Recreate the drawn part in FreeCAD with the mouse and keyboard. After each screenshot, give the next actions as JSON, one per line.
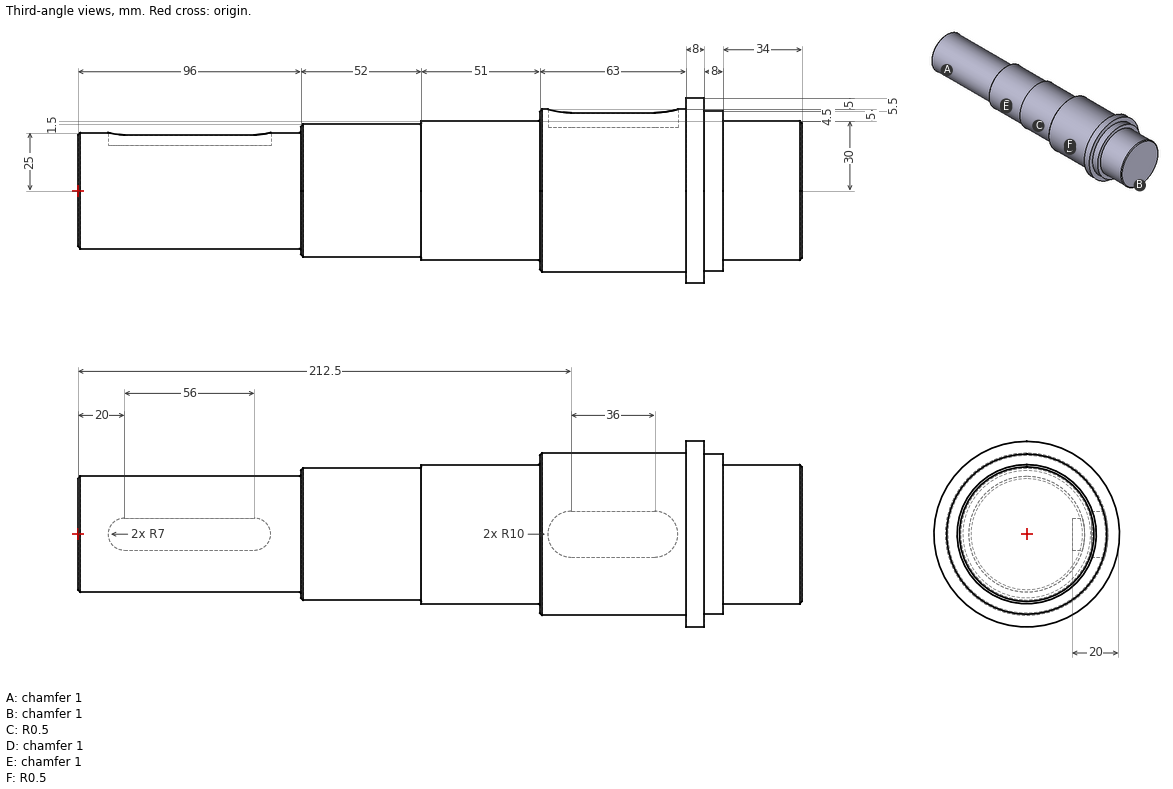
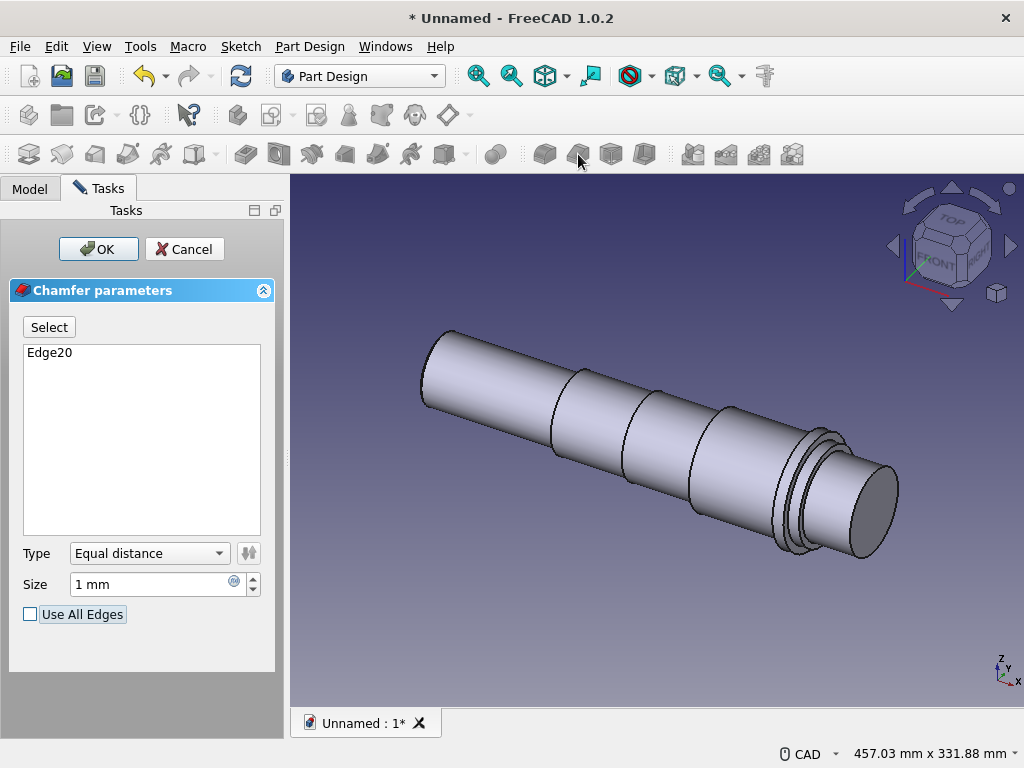
{"action": "left_click", "coordinate": [99, 249]}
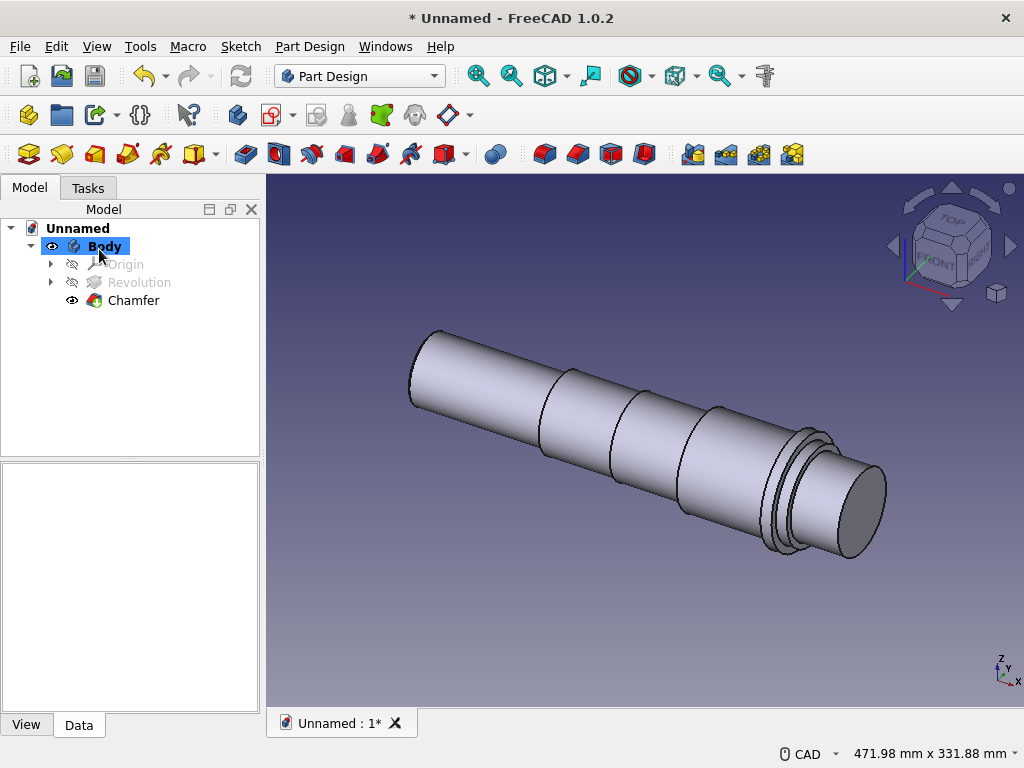
{"action": "left_click", "coordinate": [838, 535]}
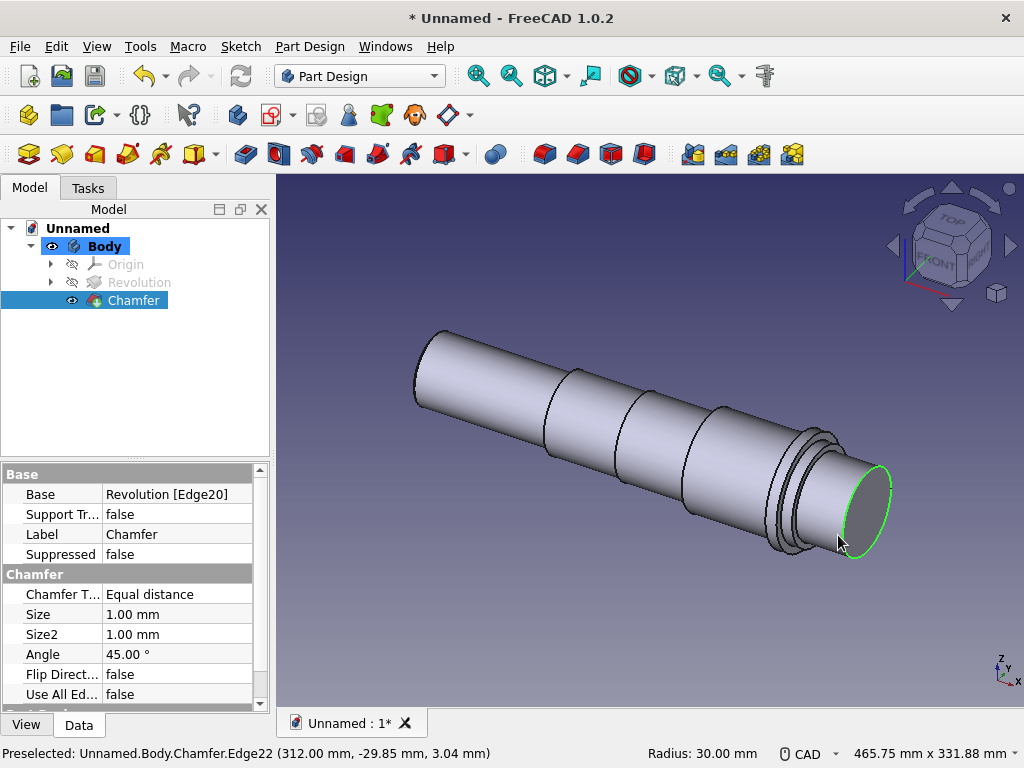
{"action": "left_click", "coordinate": [578, 154]}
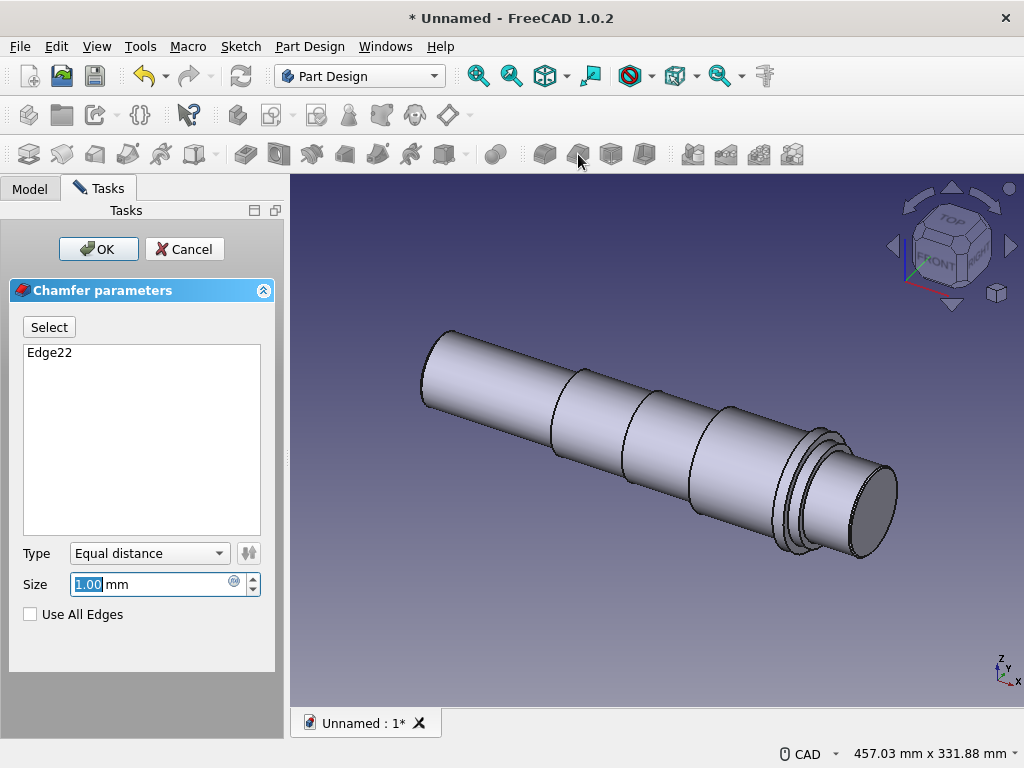
{"action": "type", "text": "1"}
{"action": "key", "text": "Tab"}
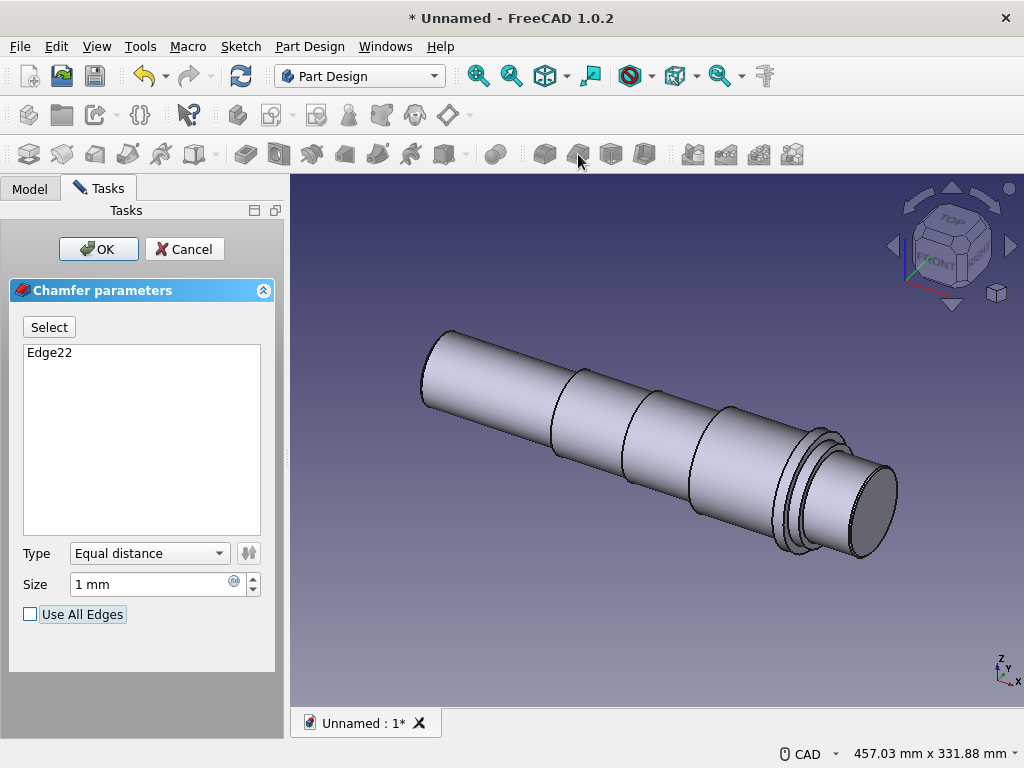
{"action": "left_click", "coordinate": [99, 249]}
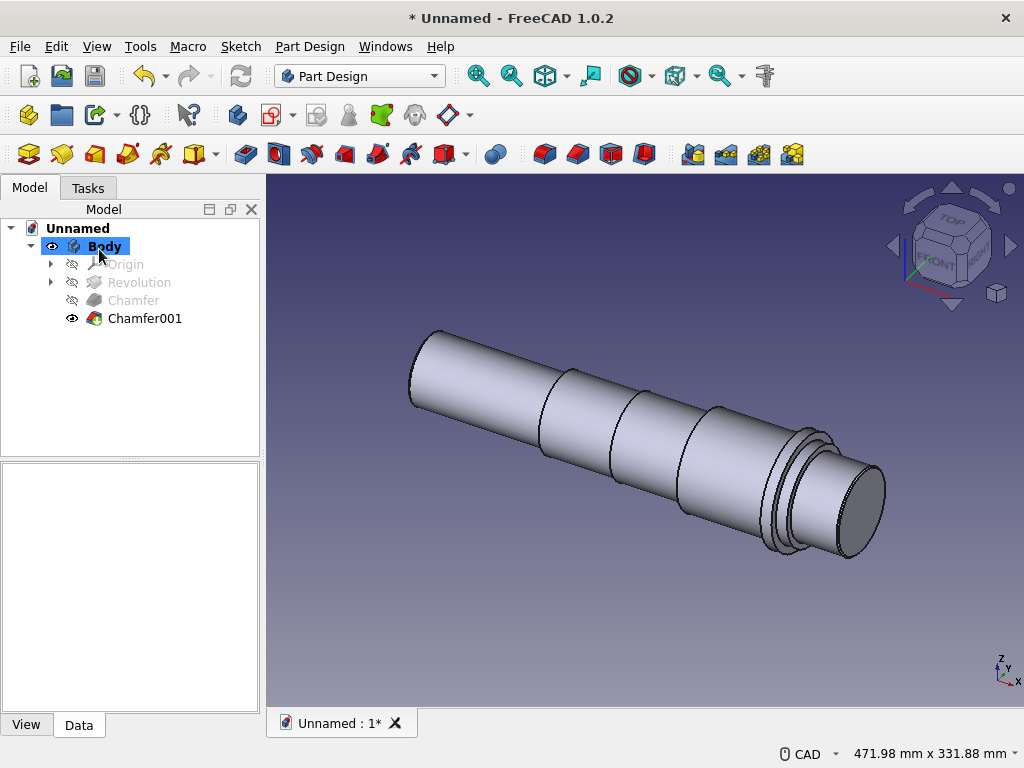
{"action": "key", "text": "0"}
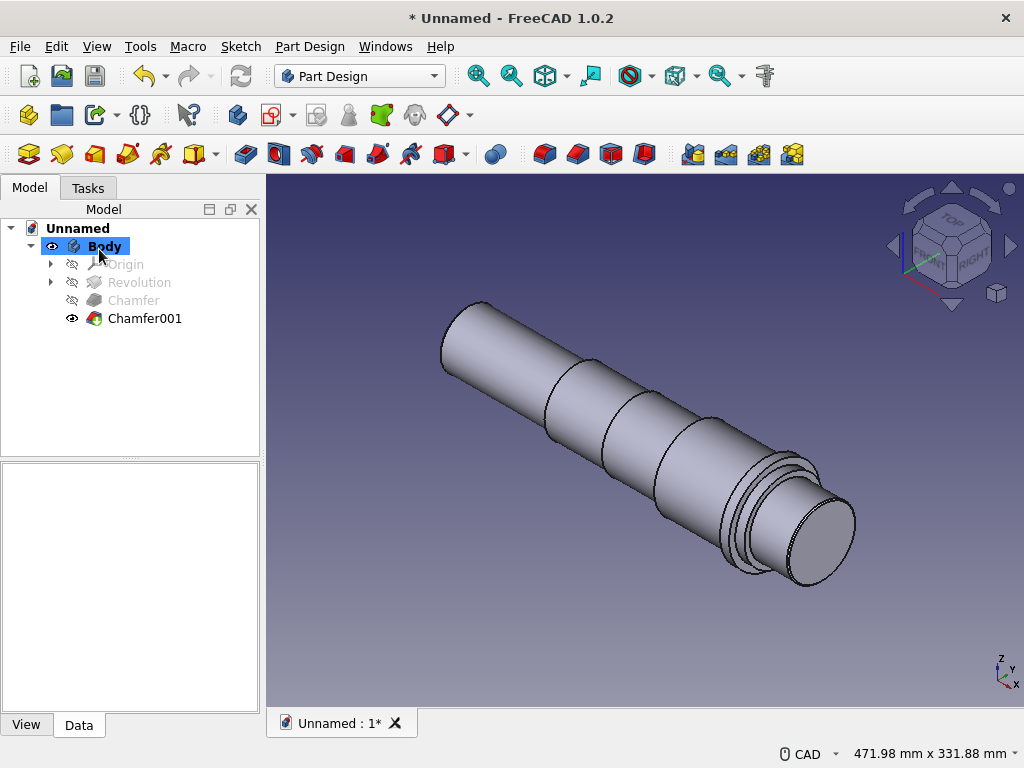
{"action": "key", "text": "2"}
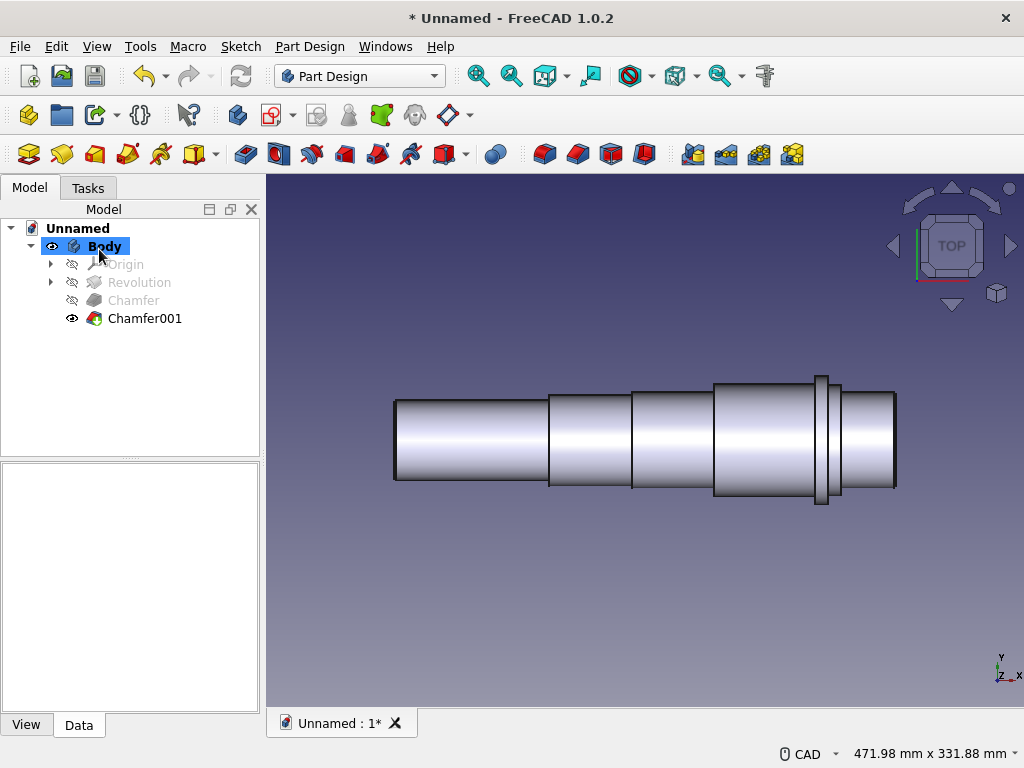
{"action": "key", "text": "1"}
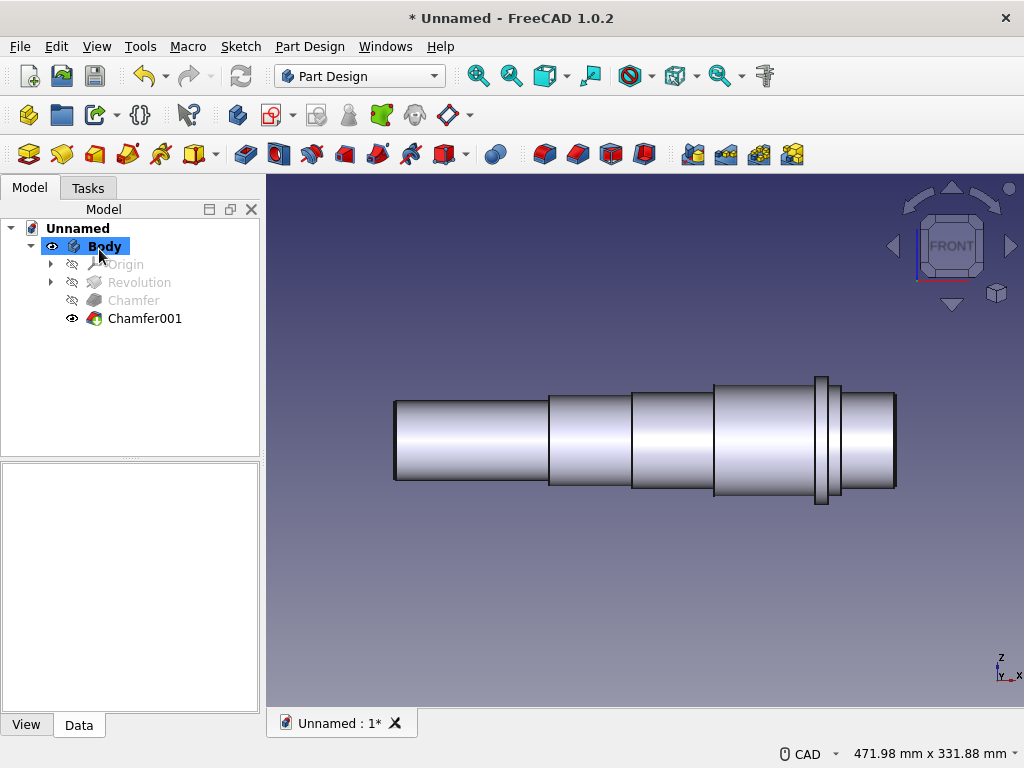
{"action": "key", "text": "3"}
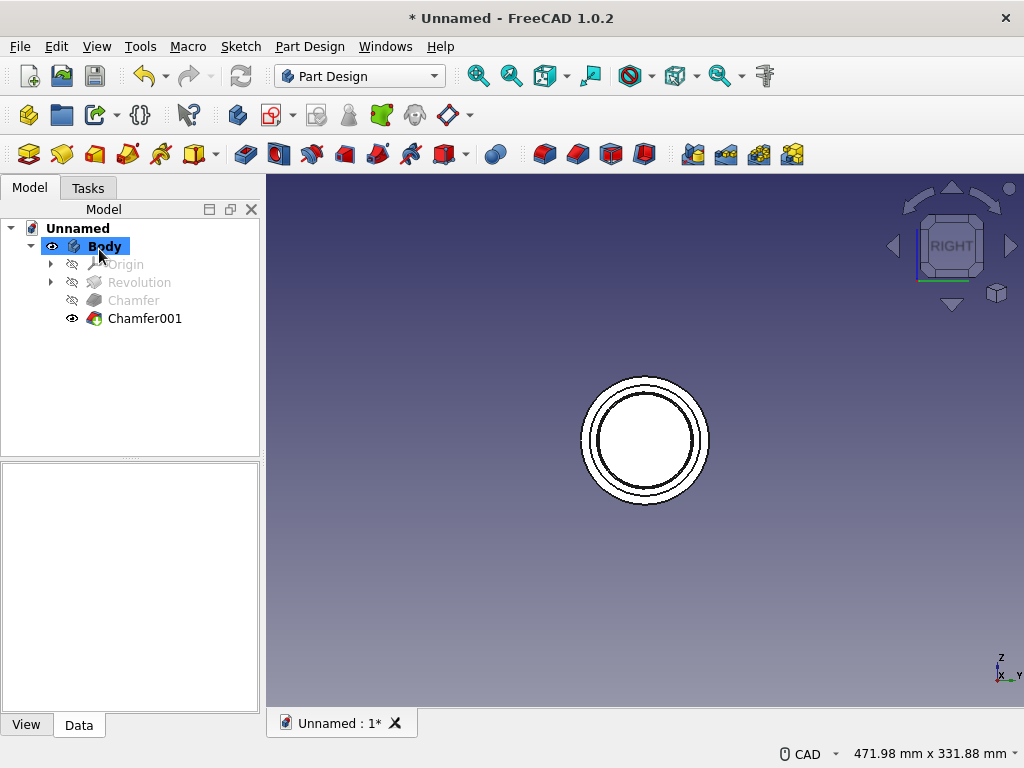
{"action": "key", "text": "v f"}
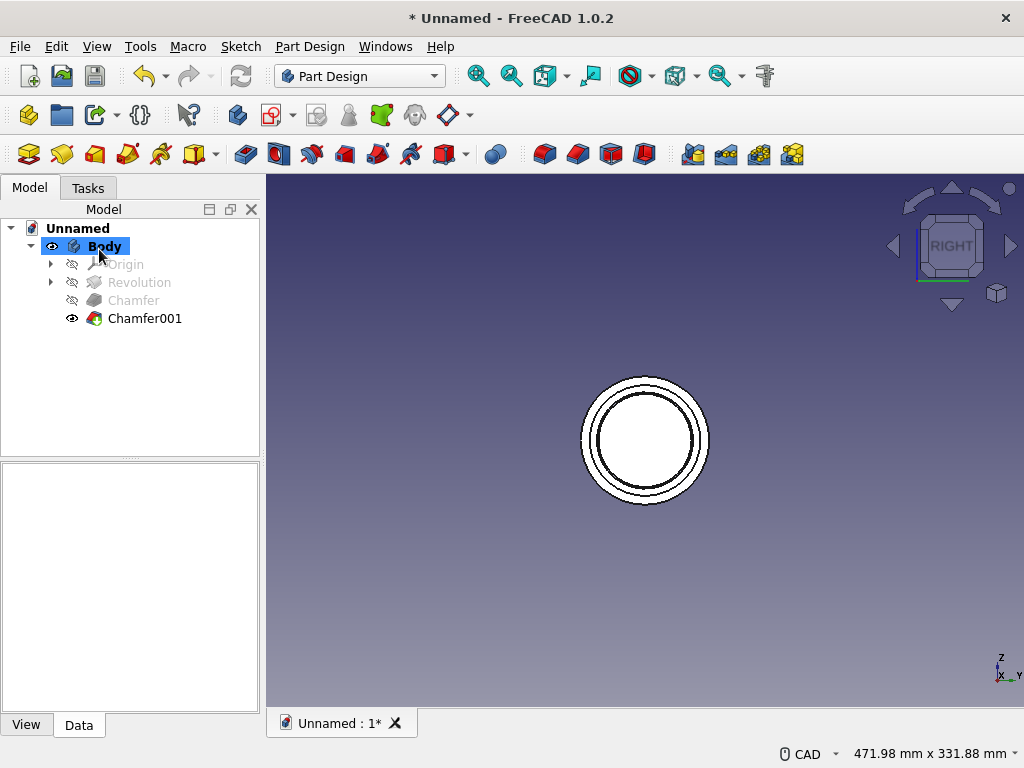
{"action": "key", "text": "5"}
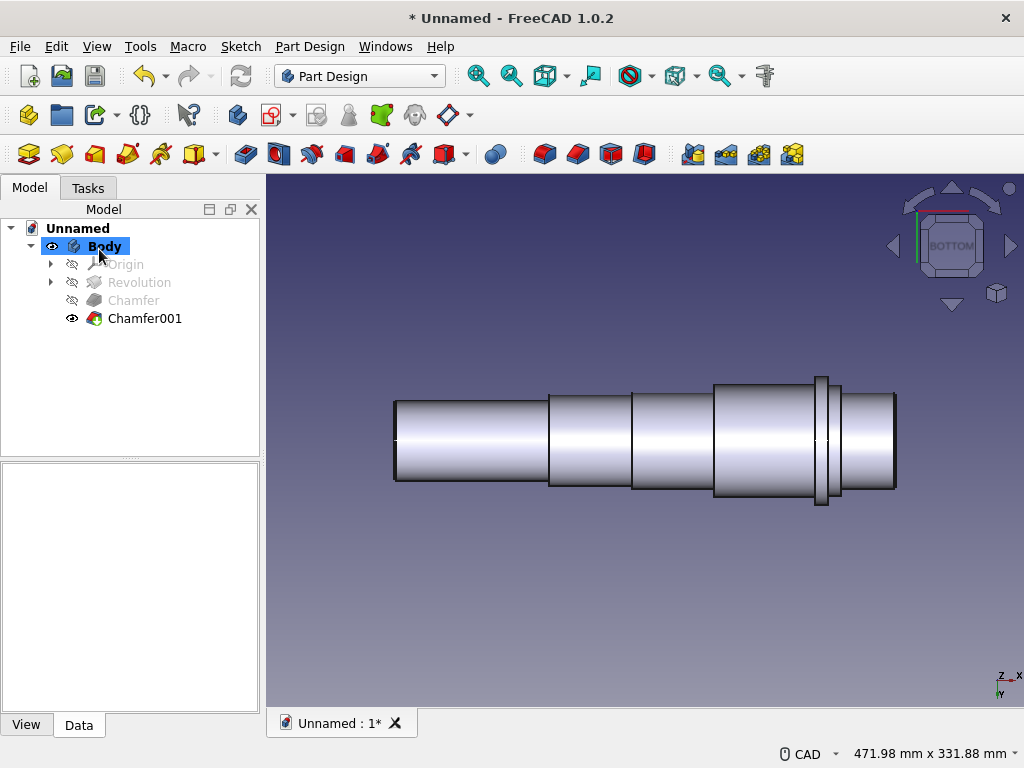
{"action": "key", "text": "4"}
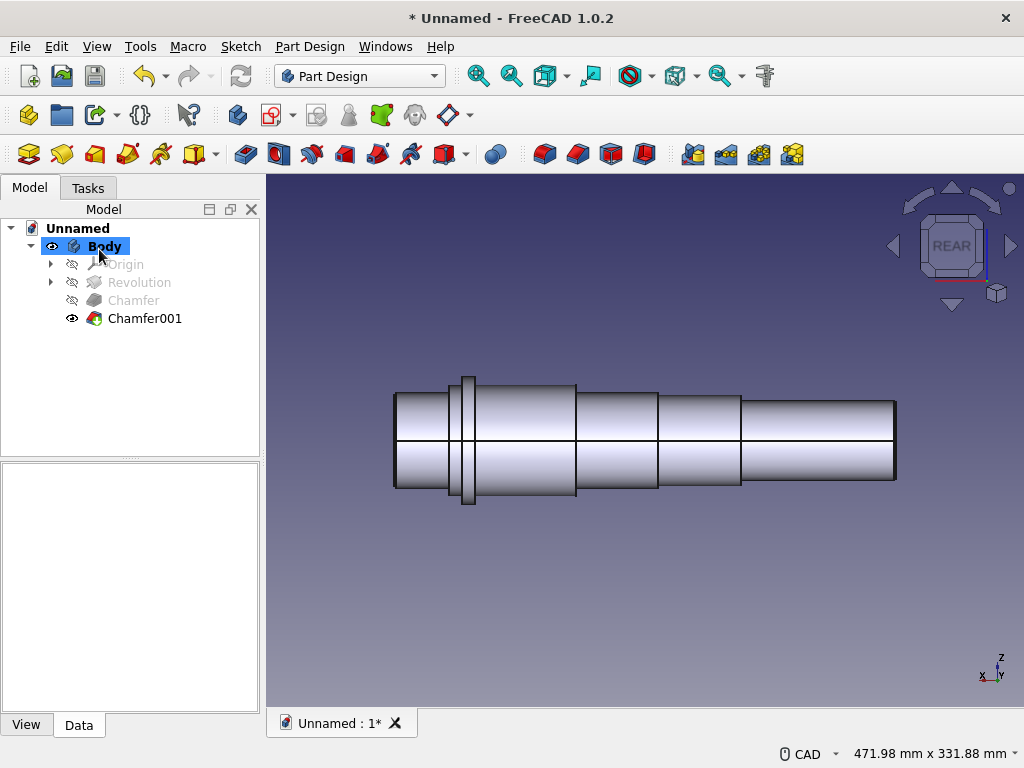
{"action": "key", "text": "6"}